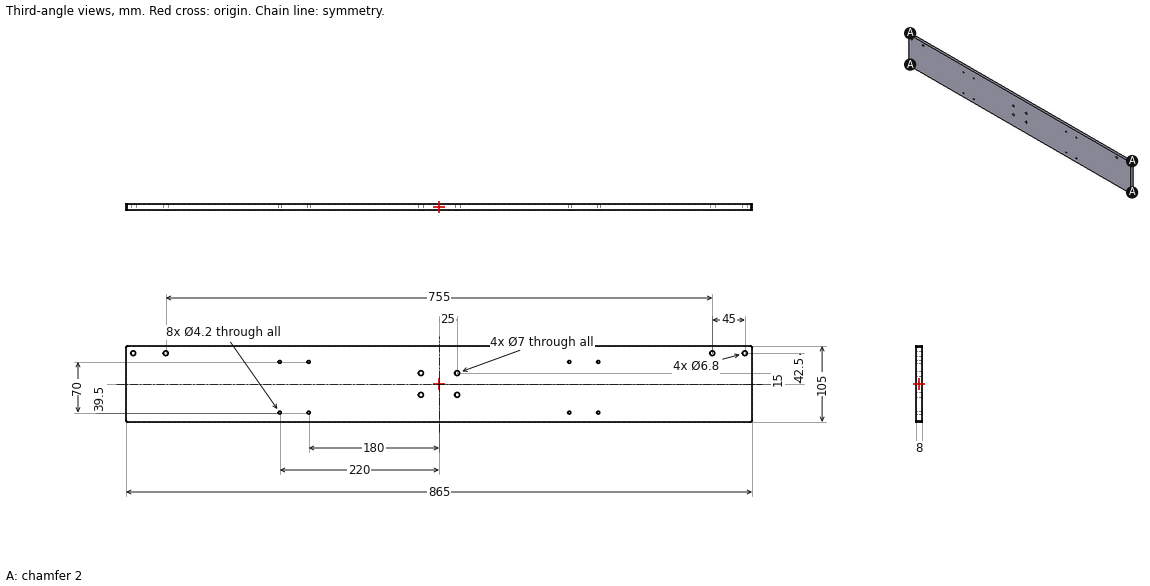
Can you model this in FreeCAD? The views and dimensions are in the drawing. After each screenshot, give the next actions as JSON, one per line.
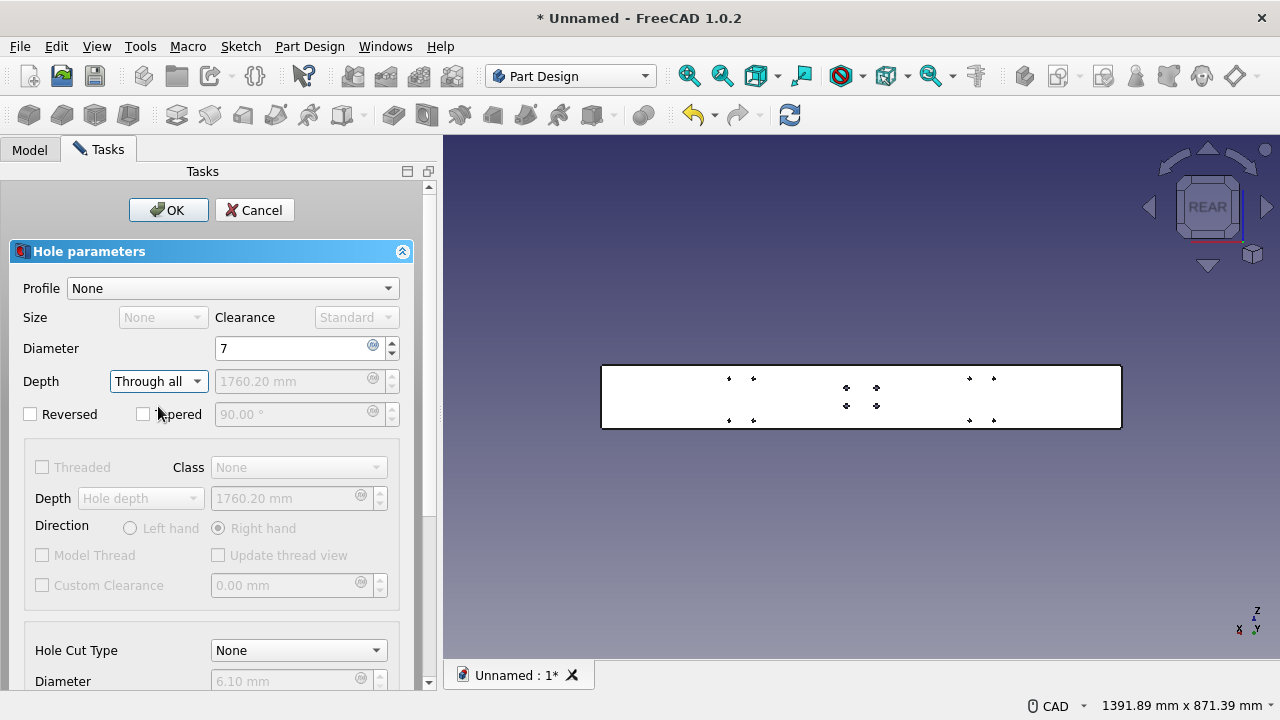
{"action": "left_click", "coordinate": [169, 210]}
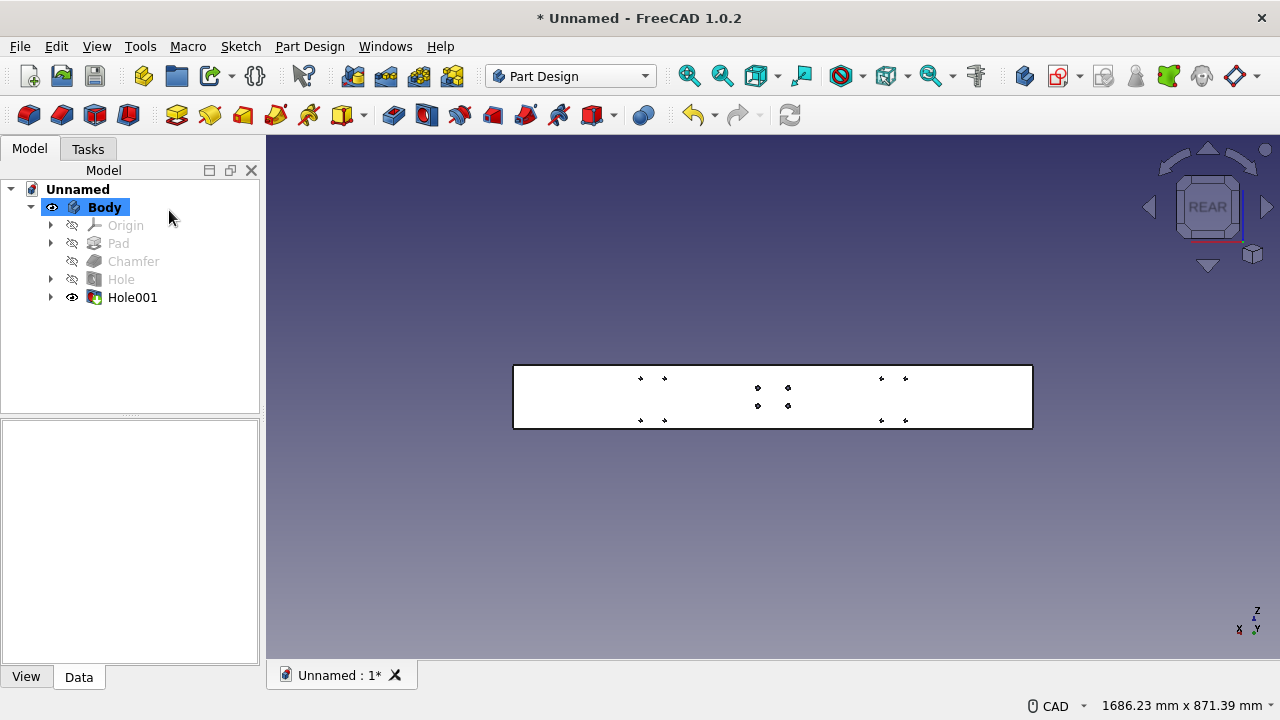
{"action": "left_click", "coordinate": [550, 396]}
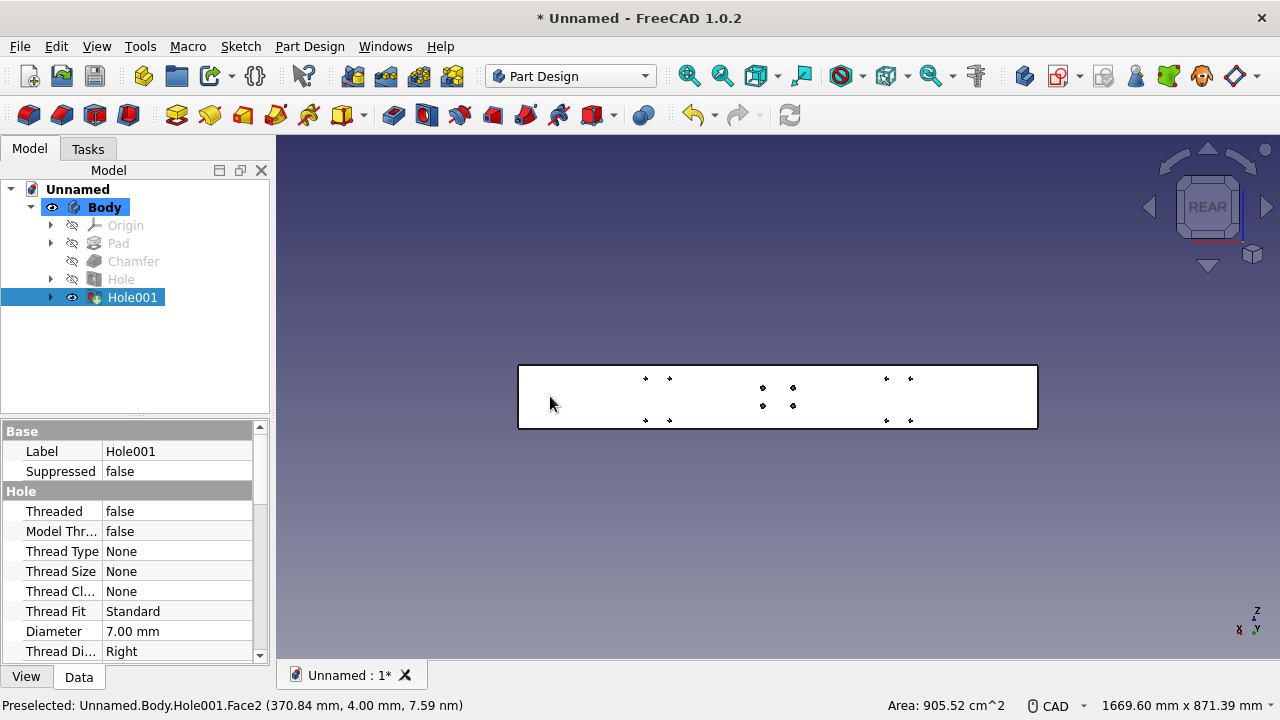
{"action": "left_click", "coordinate": [1058, 76]}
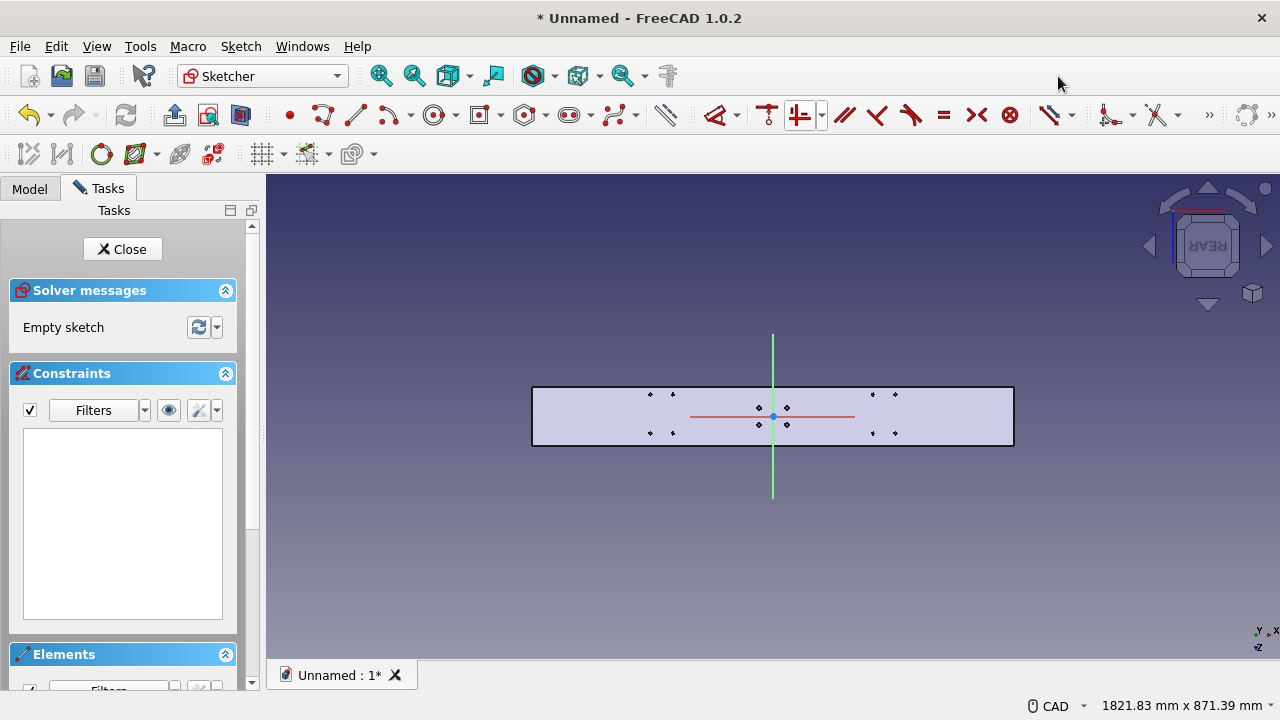
{"action": "key", "text": "g c"}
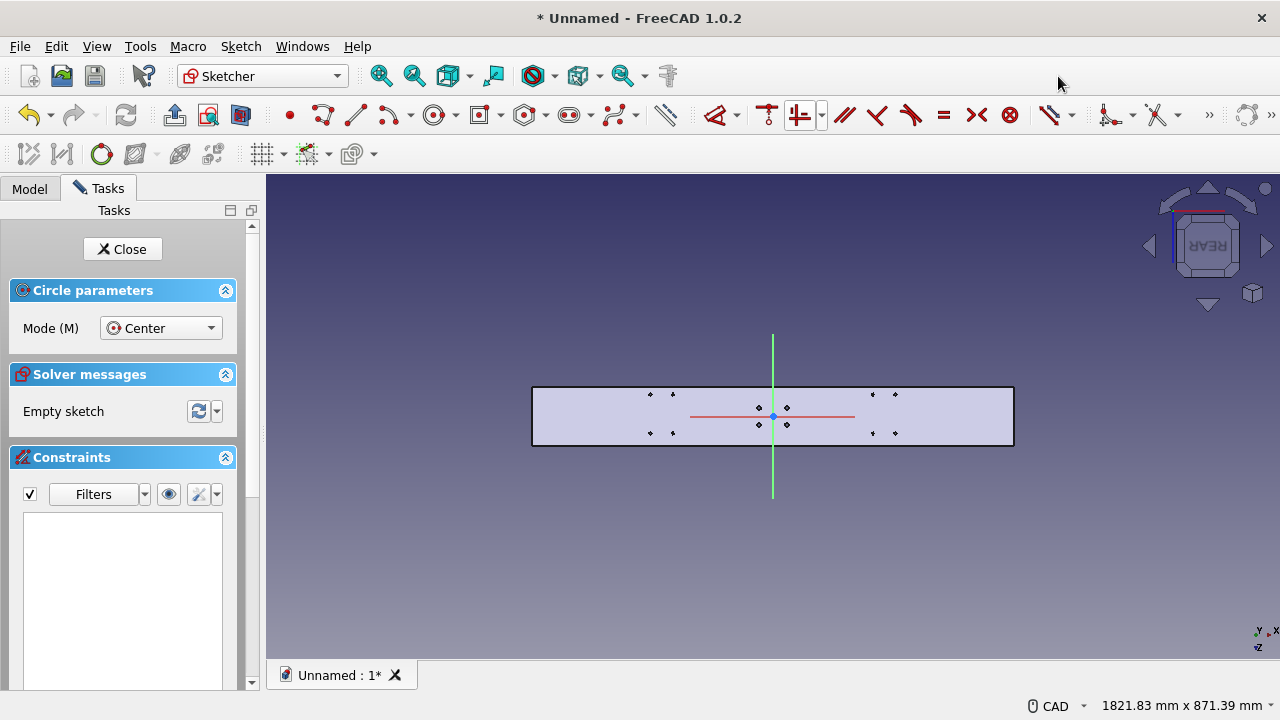
{"action": "scroll", "coordinate": [1008, 440], "scroll_direction": "up", "scroll_amount": 13}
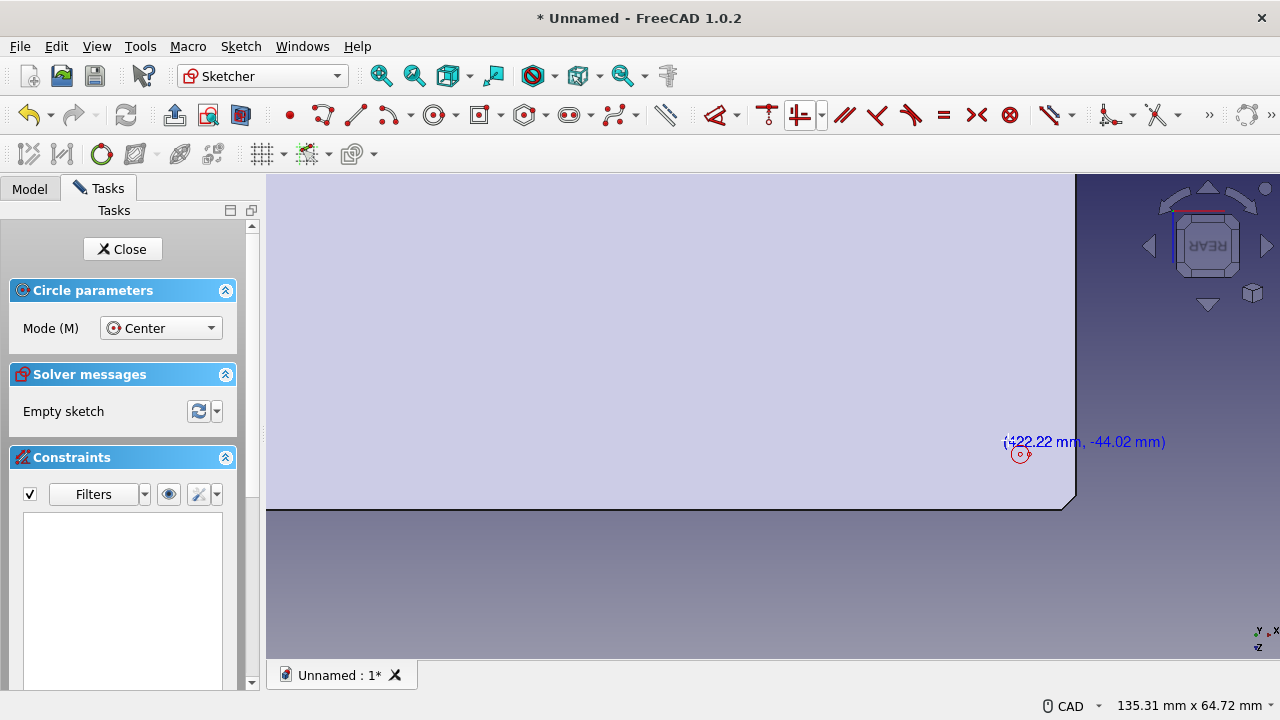
{"action": "scroll", "coordinate": [991, 429], "scroll_direction": "down", "scroll_amount": 12}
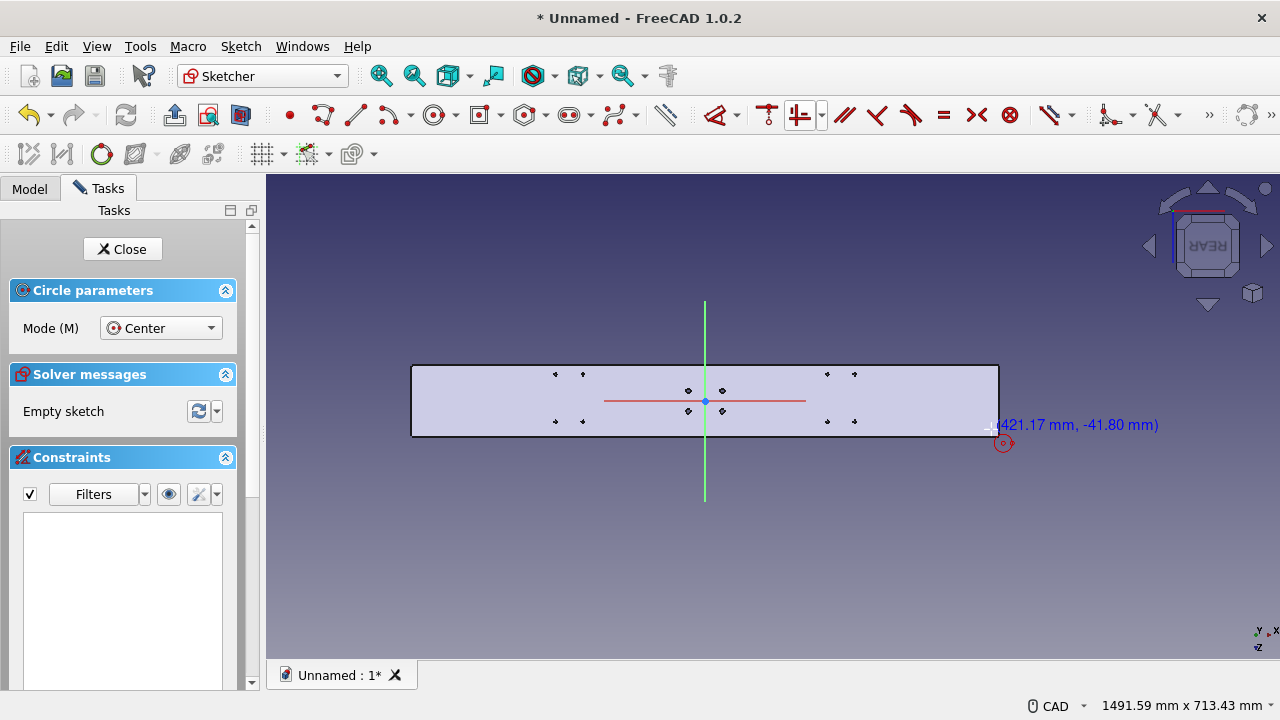
{"action": "left_click", "coordinate": [993, 430]}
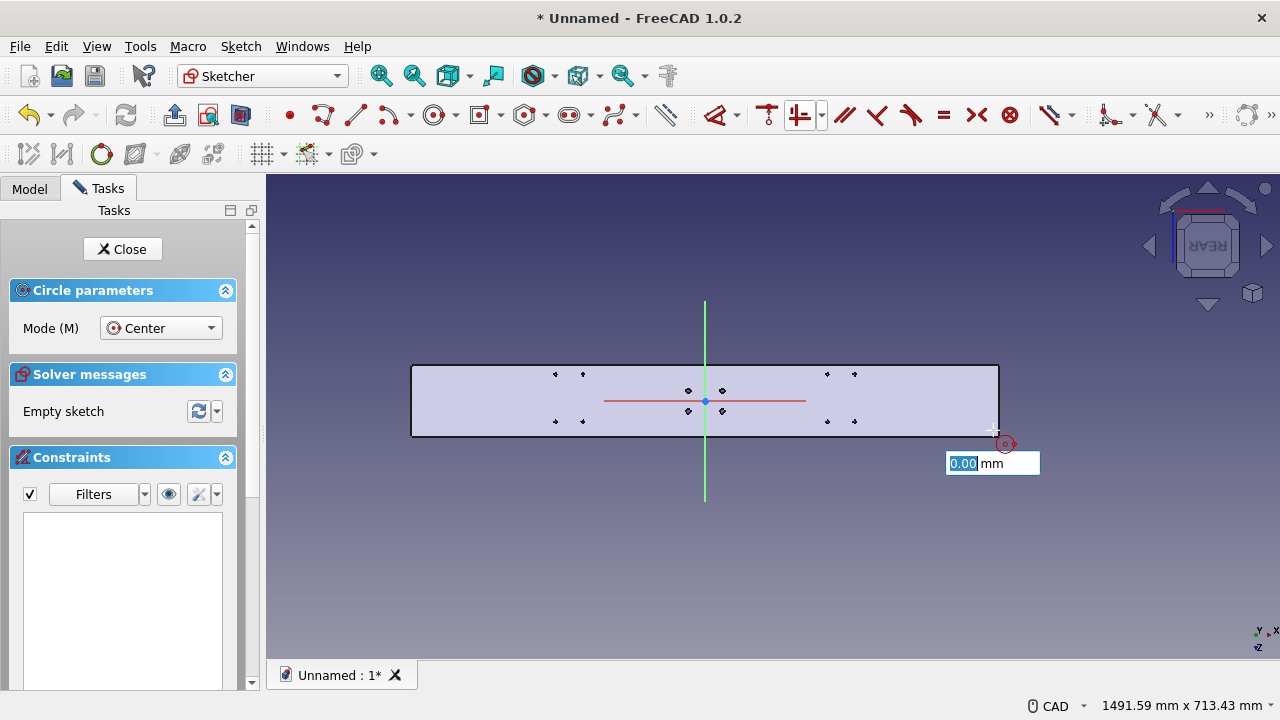
{"action": "scroll", "coordinate": [994, 428], "scroll_direction": "up", "scroll_amount": 10}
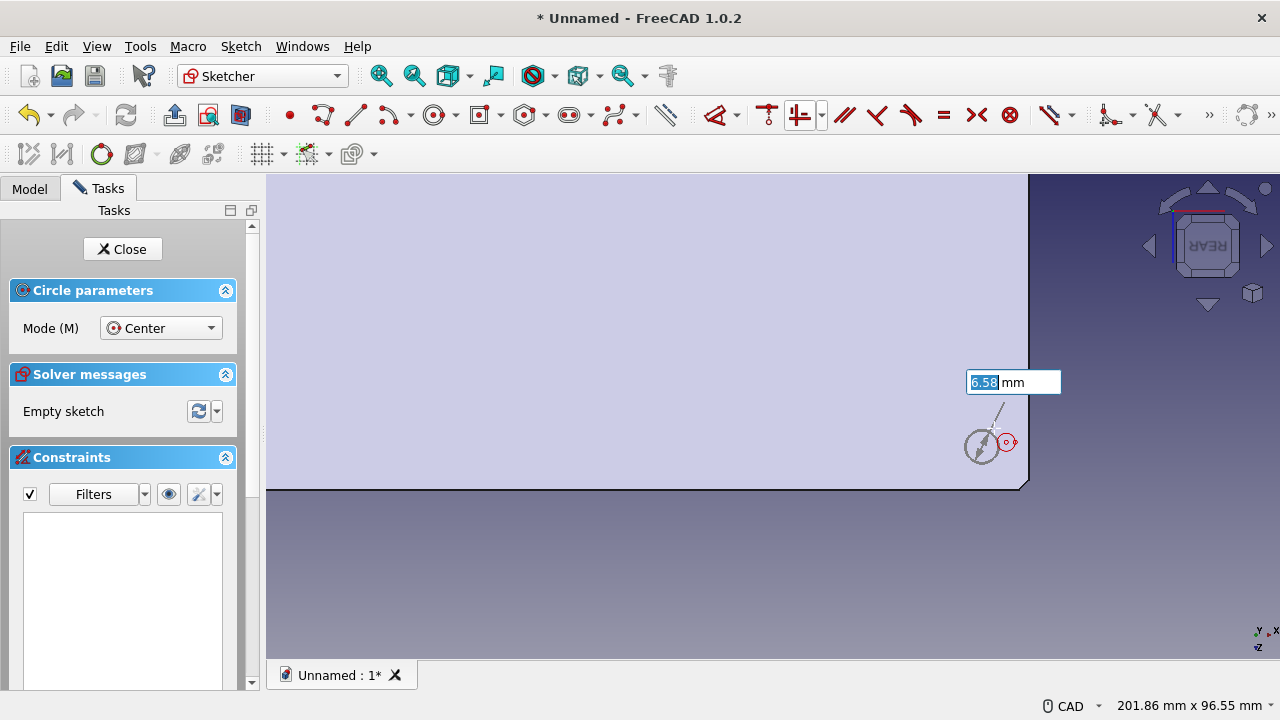
{"action": "left_click", "coordinate": [991, 428]}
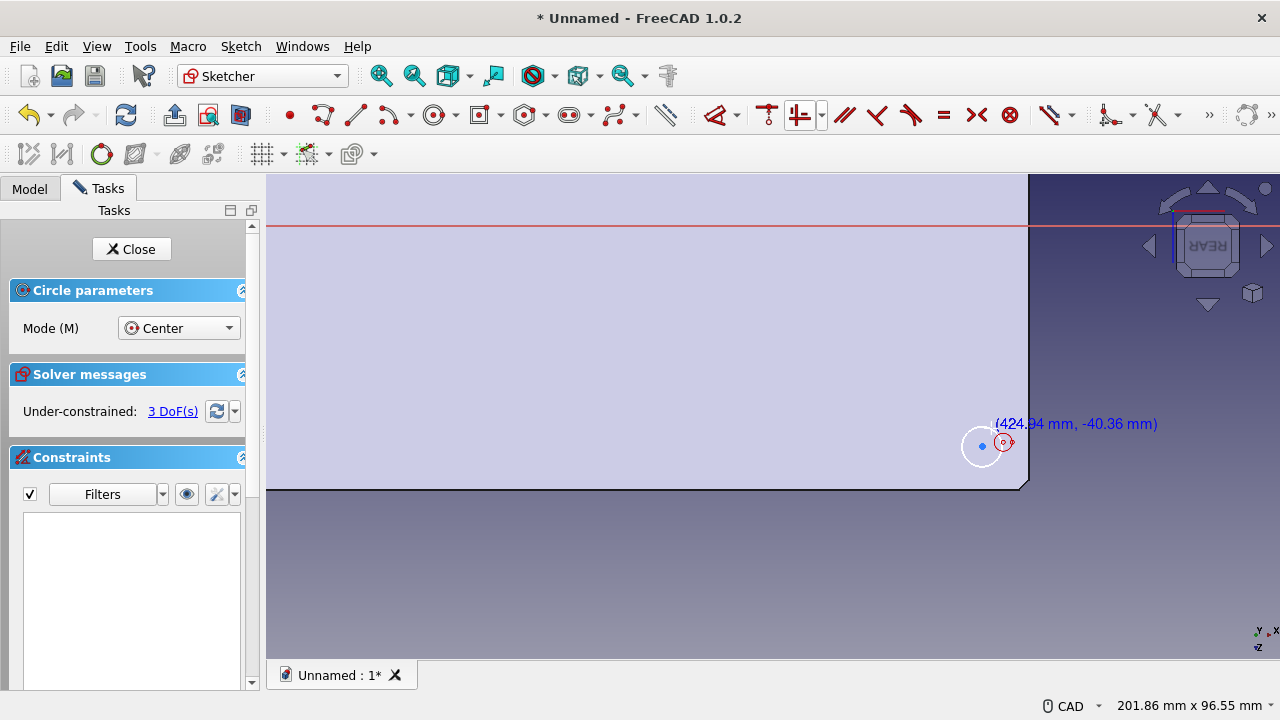
{"action": "scroll", "coordinate": [753, 440], "scroll_direction": "up", "scroll_amount": 2}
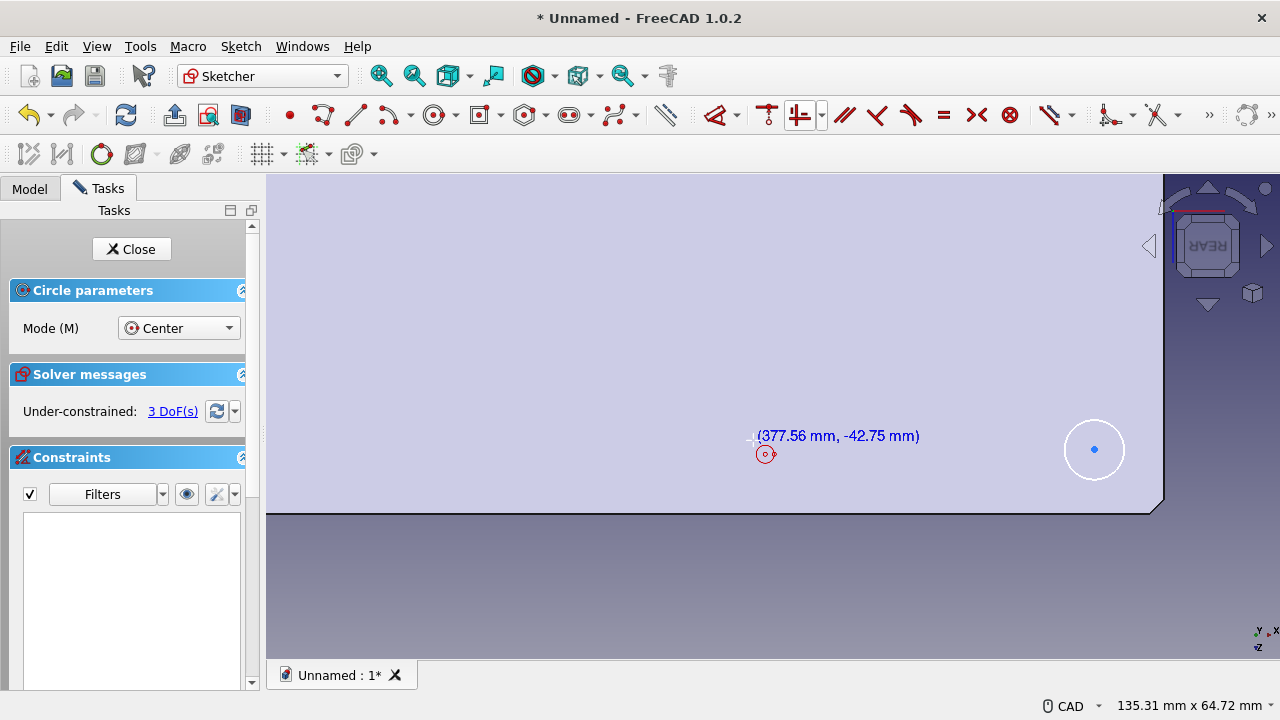
{"action": "scroll", "coordinate": [982, 429], "scroll_direction": "down", "scroll_amount": 12}